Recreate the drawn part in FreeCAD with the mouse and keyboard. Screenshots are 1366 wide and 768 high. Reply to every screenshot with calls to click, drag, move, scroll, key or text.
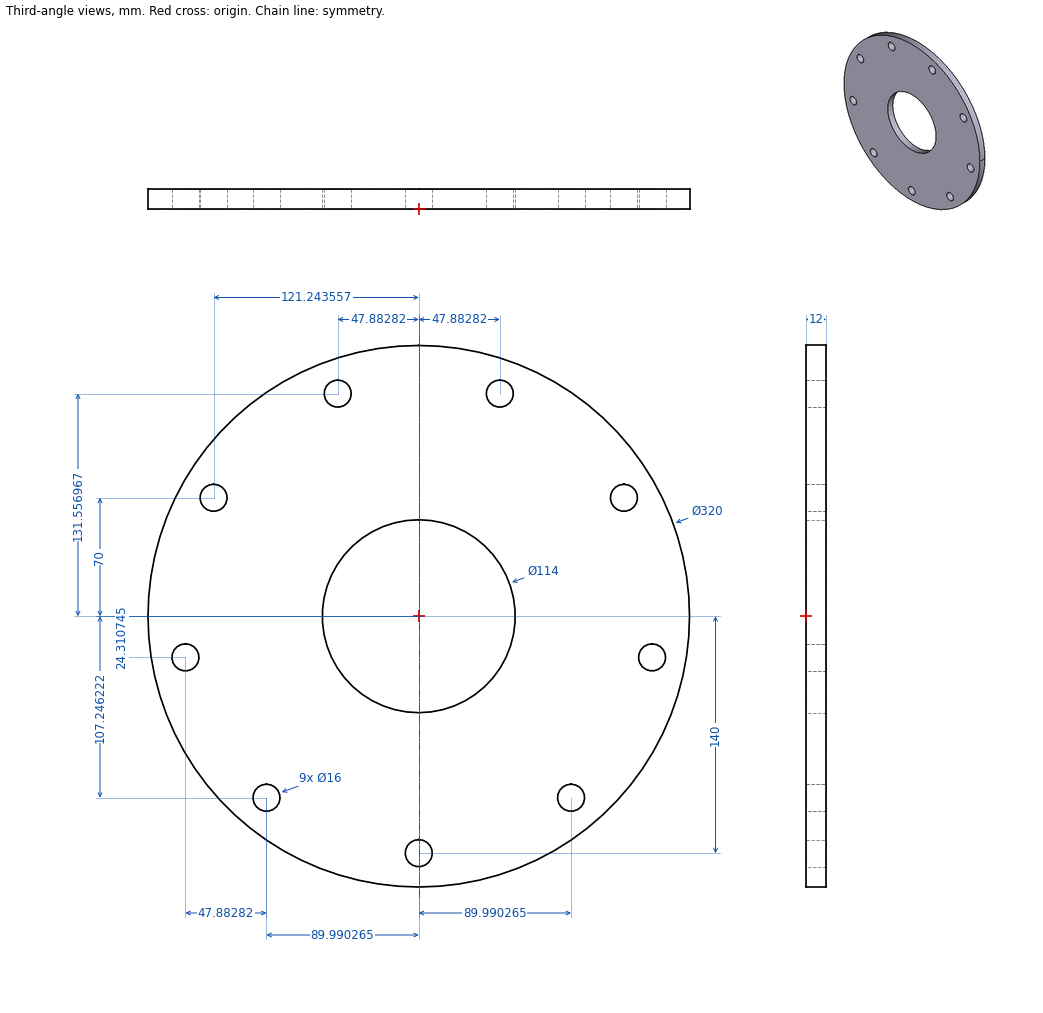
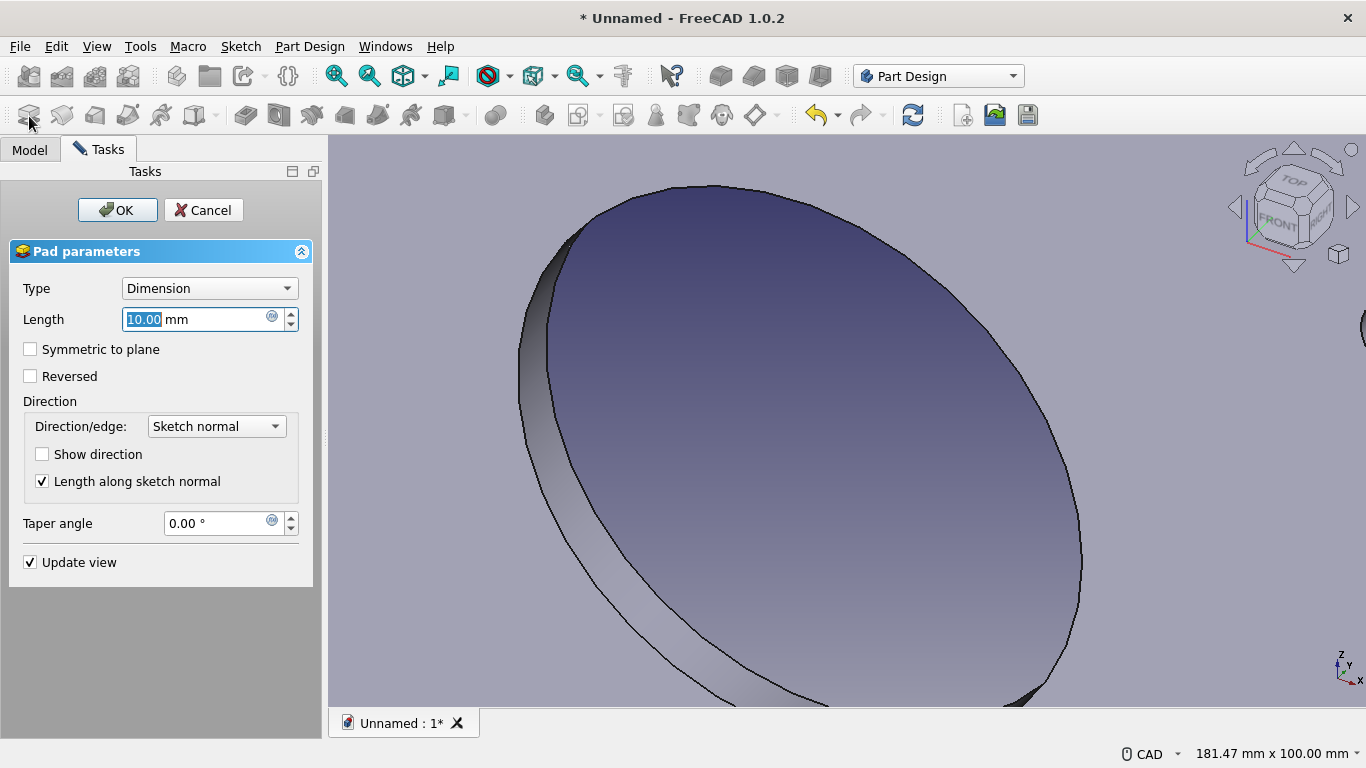
text(12)
key(Tab)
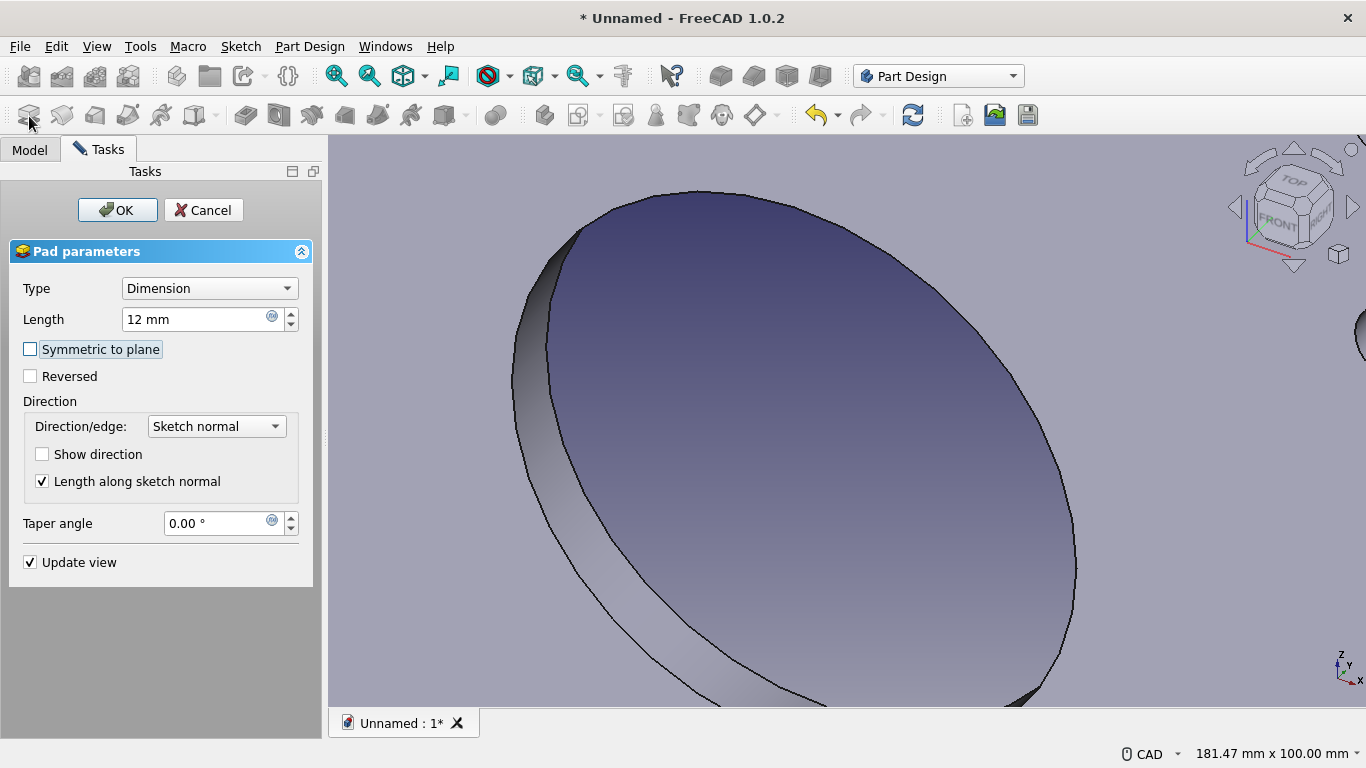
click(31, 376)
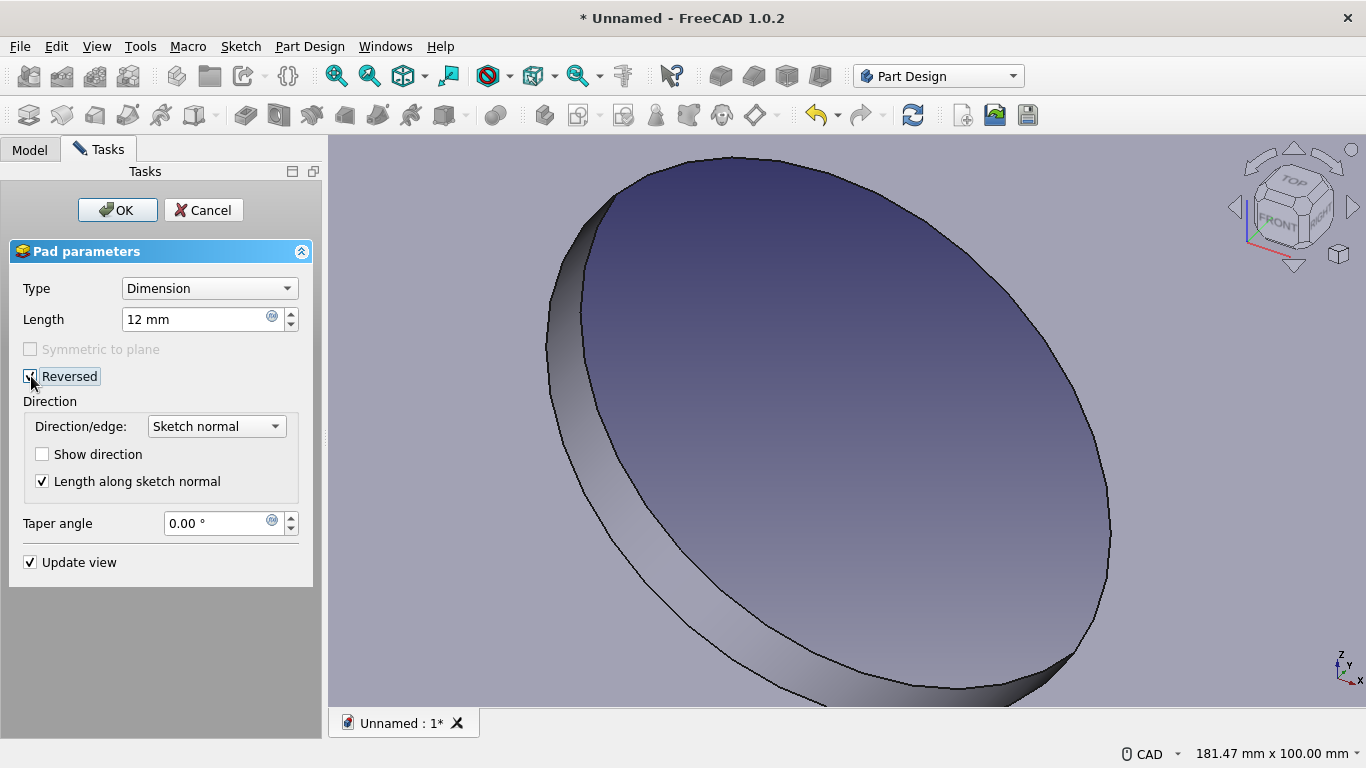
click(118, 210)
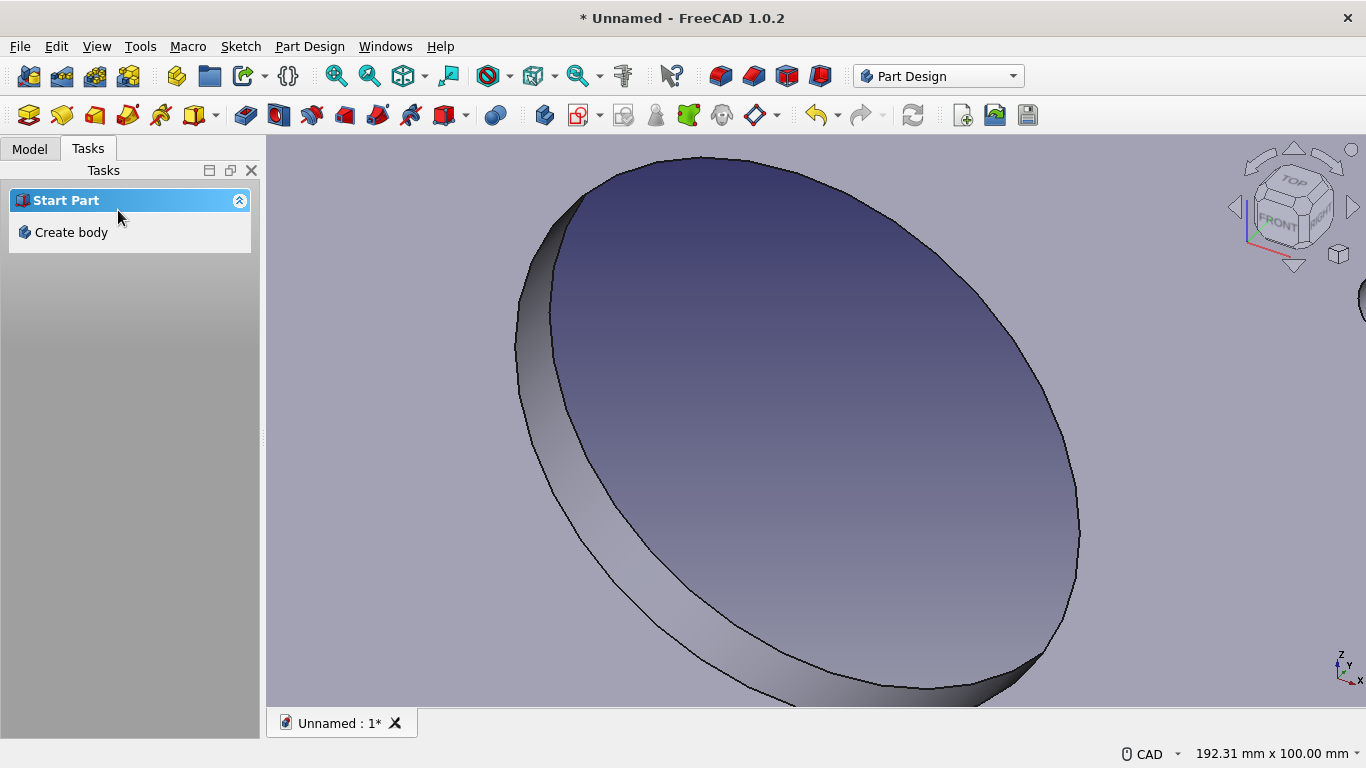
key(0)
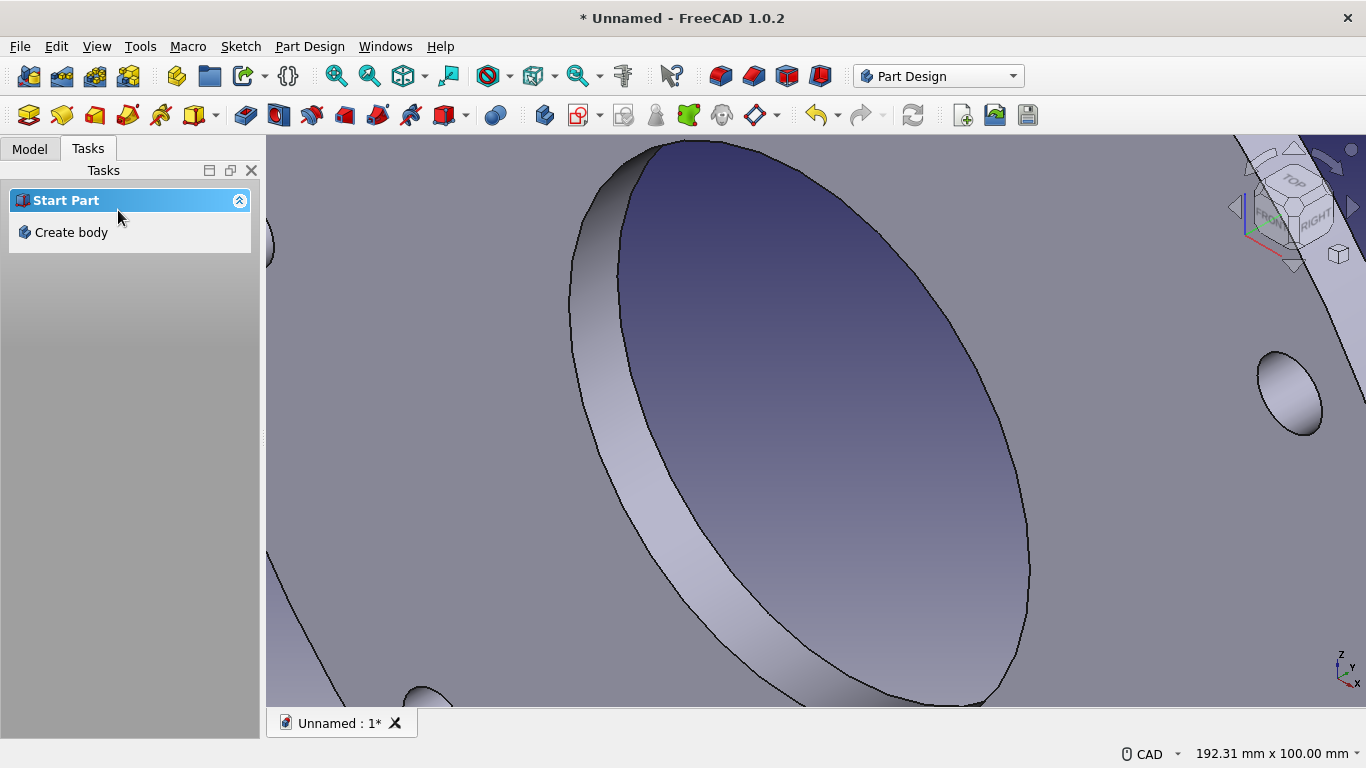
click(337, 76)